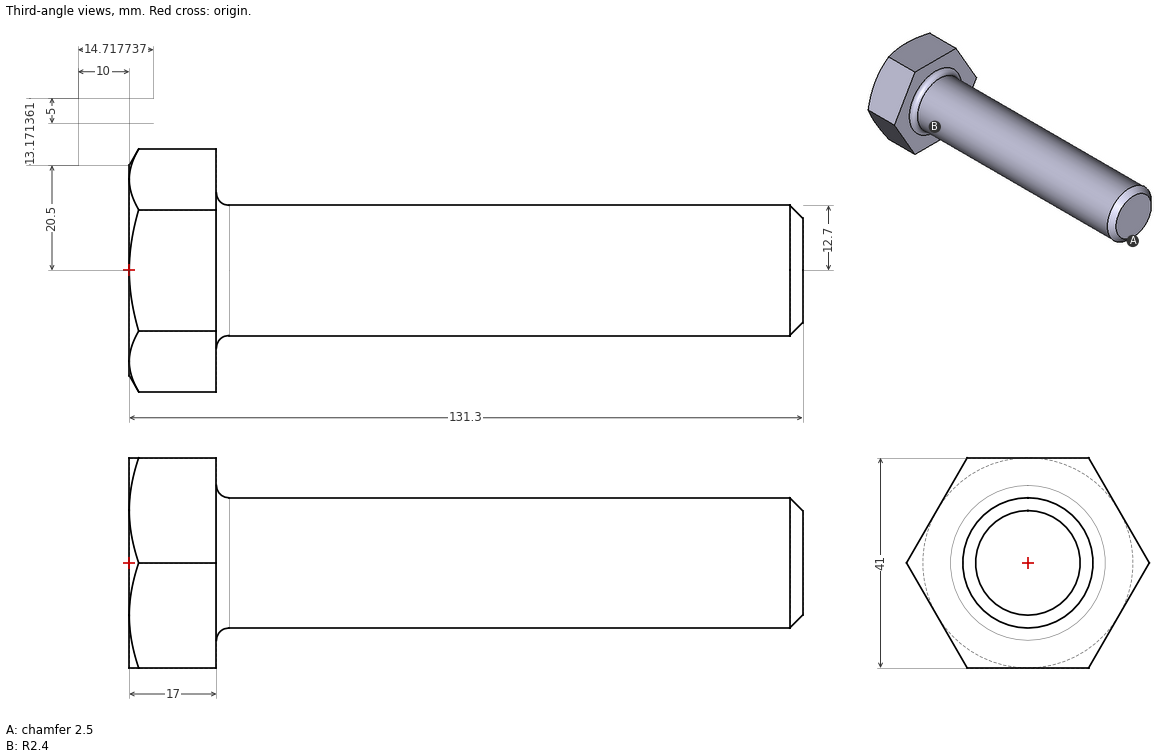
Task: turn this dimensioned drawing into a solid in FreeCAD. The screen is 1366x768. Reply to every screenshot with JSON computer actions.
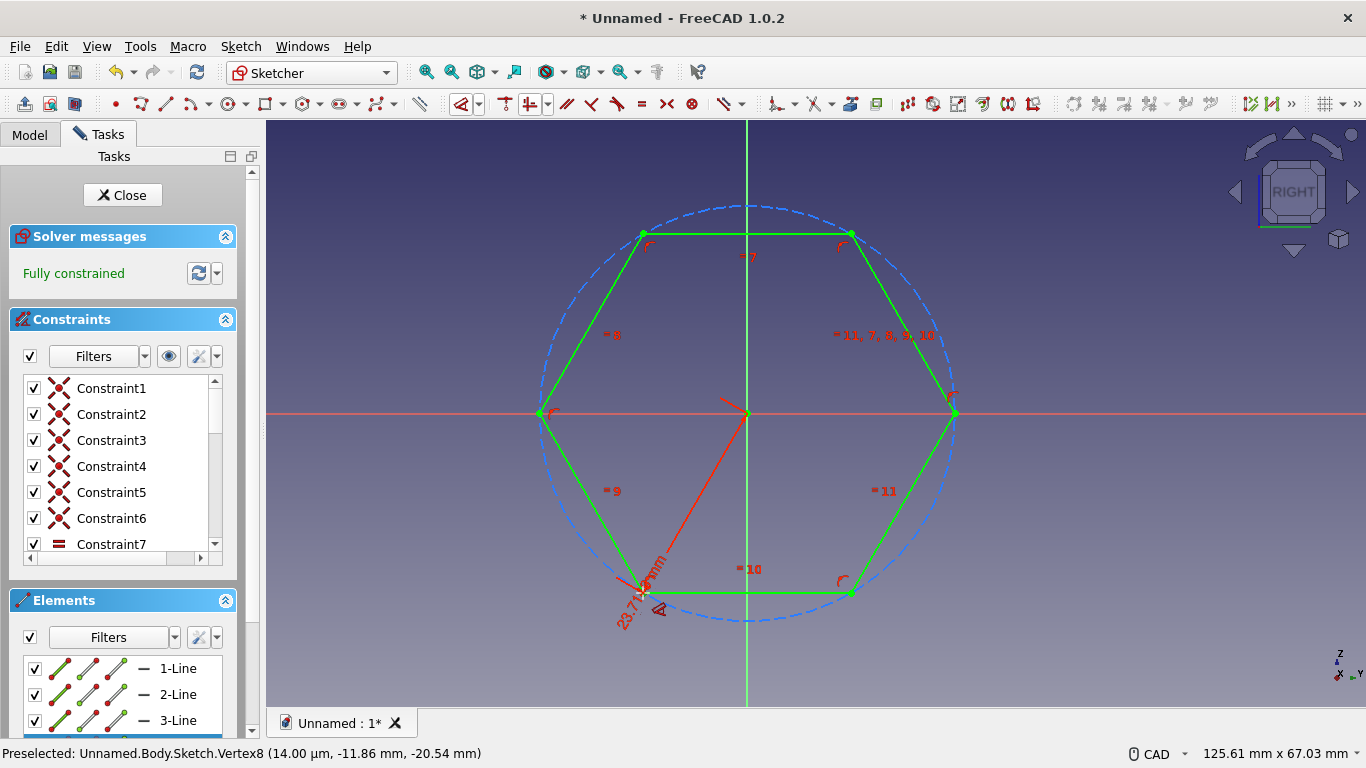
{"action": "left_click", "coordinate": [851, 234]}
{"action": "left_click", "coordinate": [885, 331]}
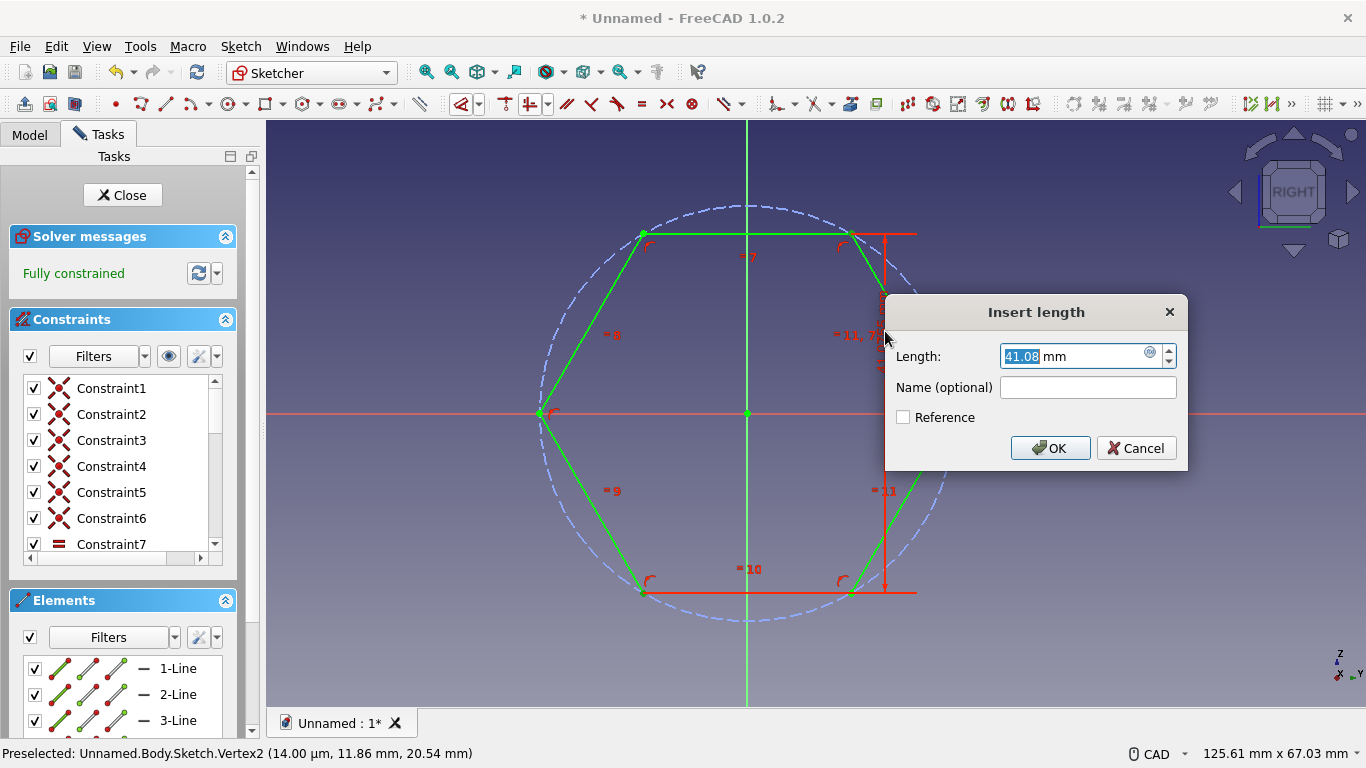
{"action": "type", "text": "41"}
{"action": "key", "text": "Return"}
{"action": "key", "text": "Escape"}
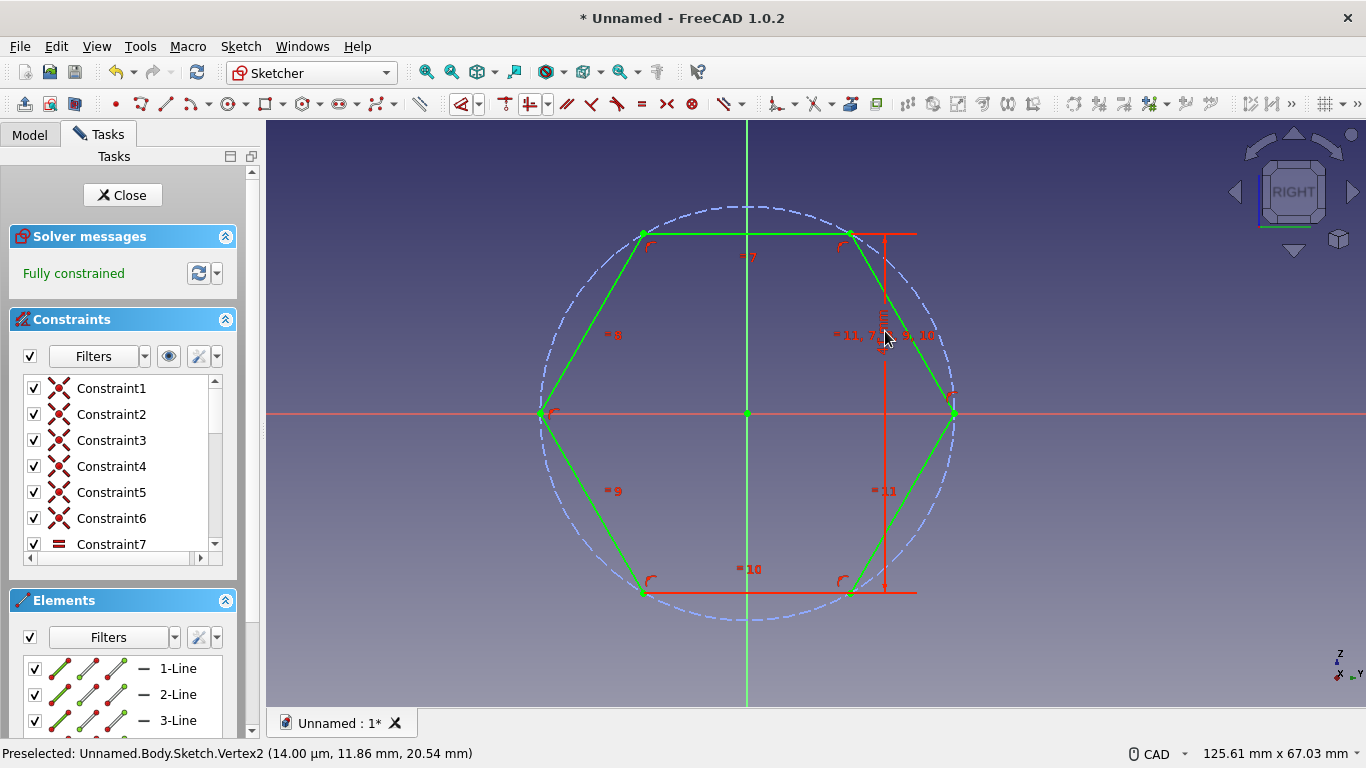
{"action": "left_click", "coordinate": [123, 195]}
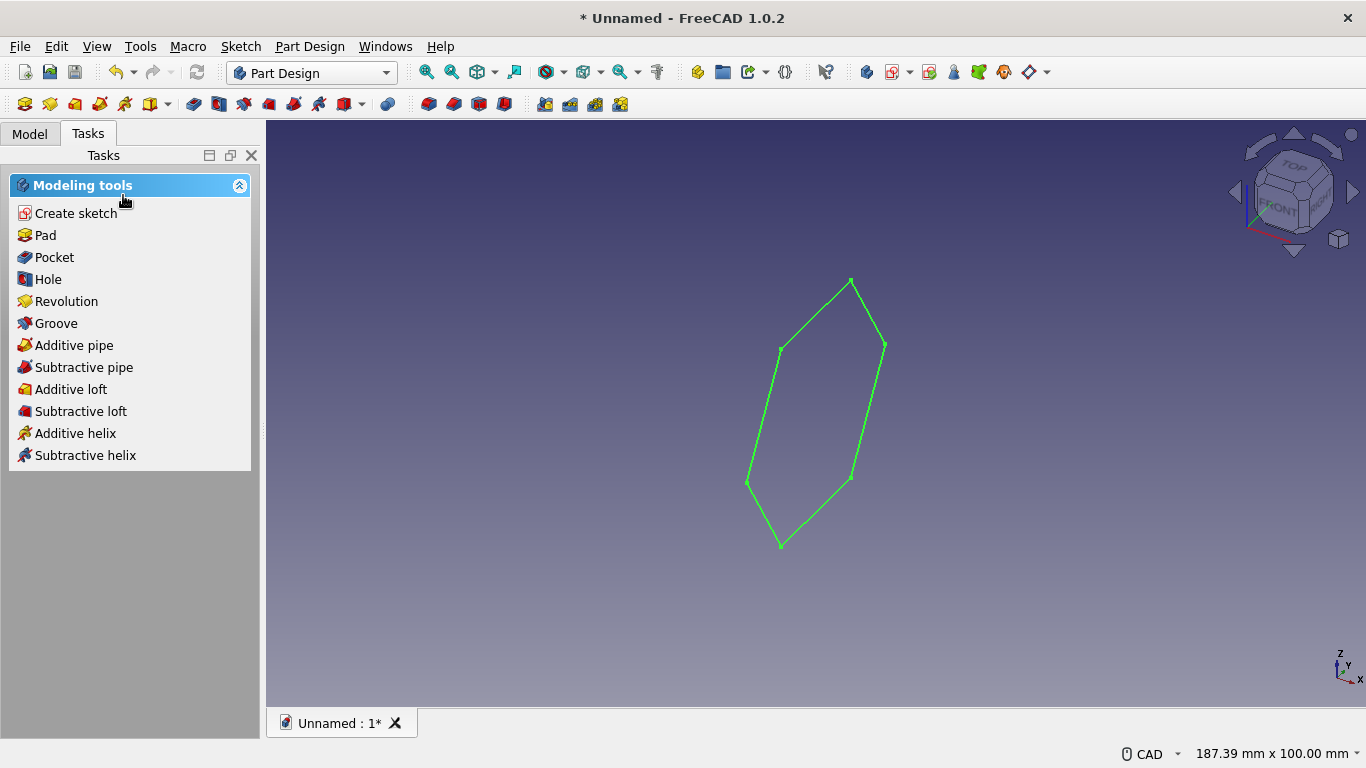
{"action": "left_click", "coordinate": [25, 104]}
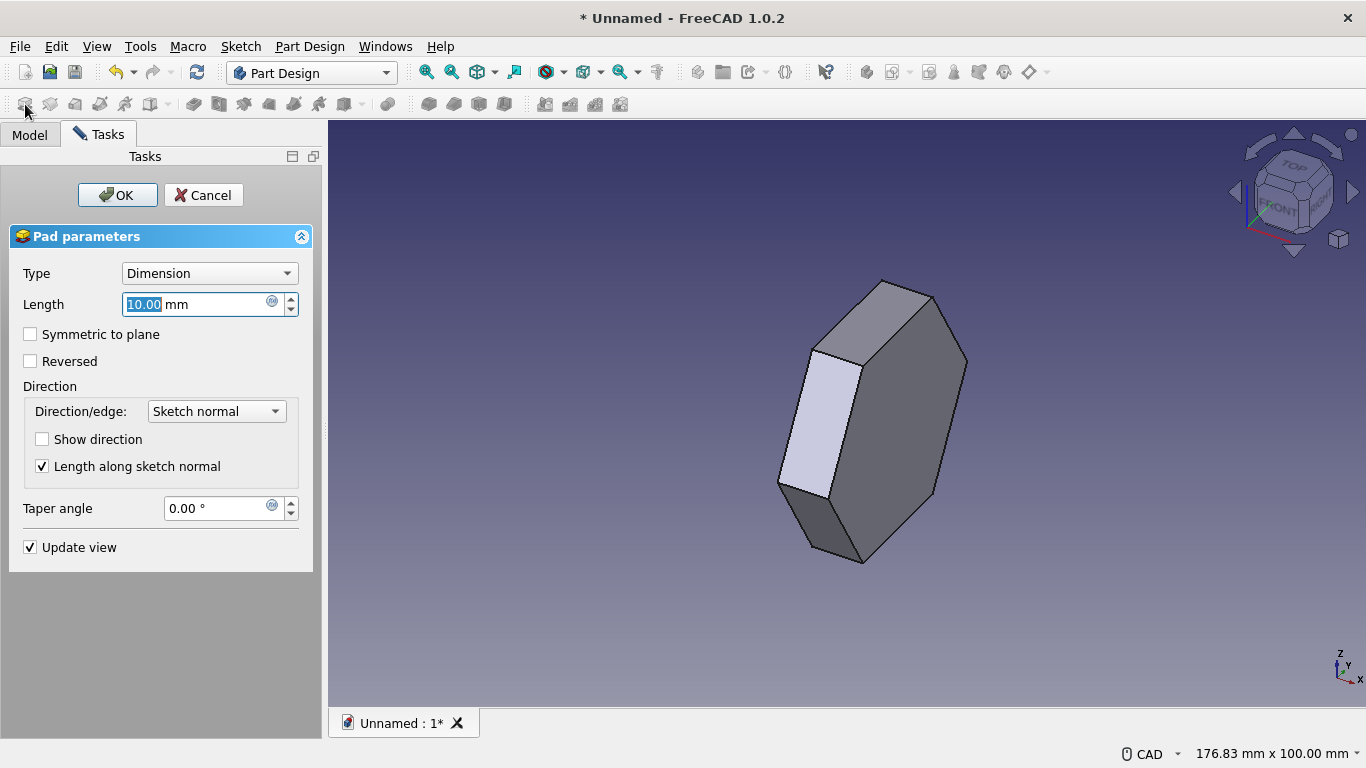
{"action": "type", "text": "17"}
{"action": "key", "text": "Tab"}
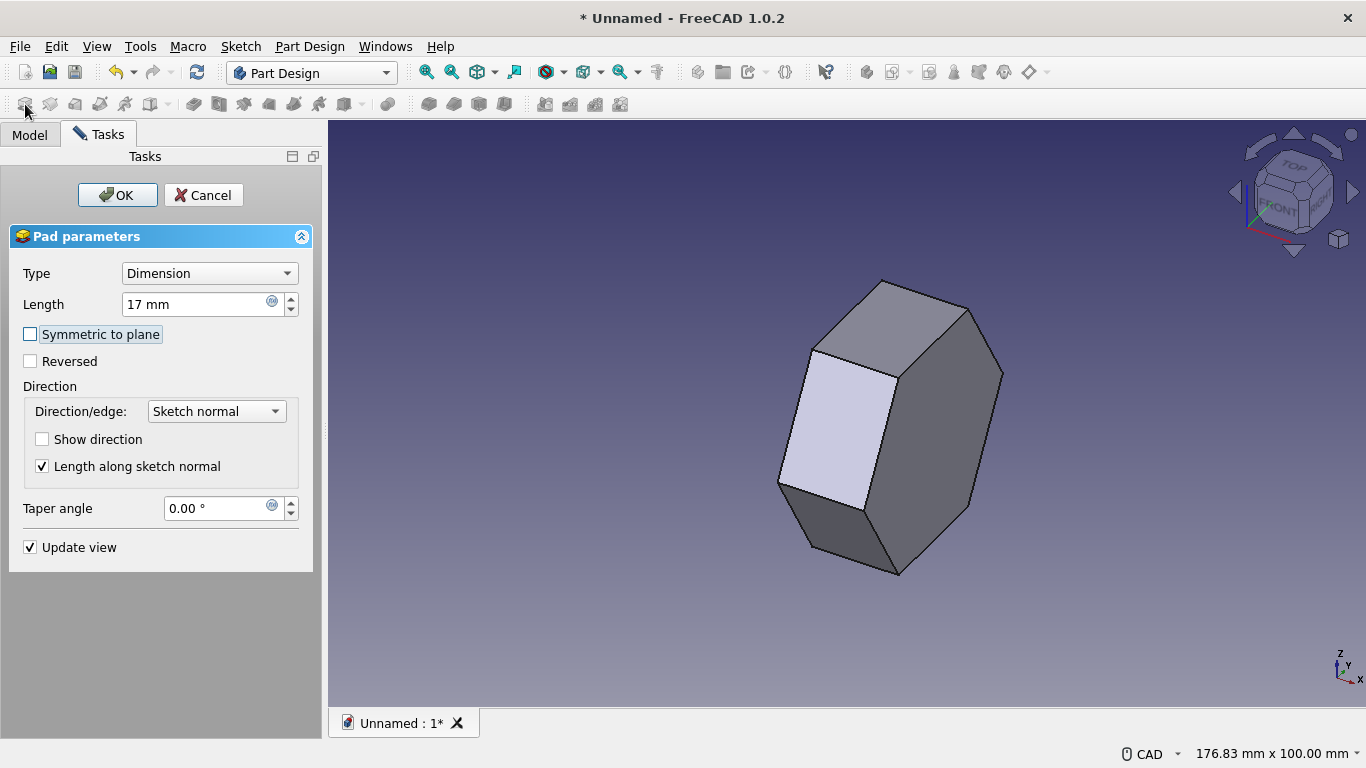
{"action": "left_click", "coordinate": [118, 195]}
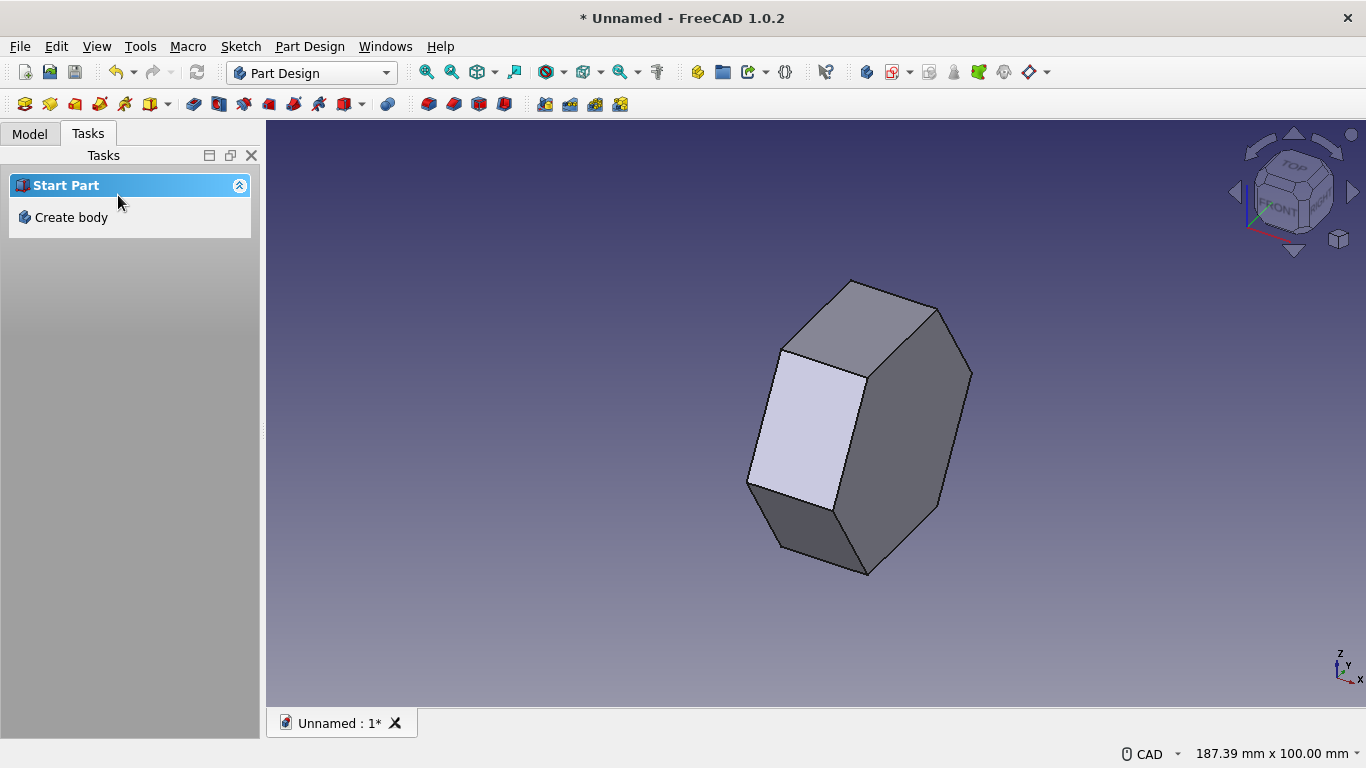
{"action": "left_click", "coordinate": [892, 72]}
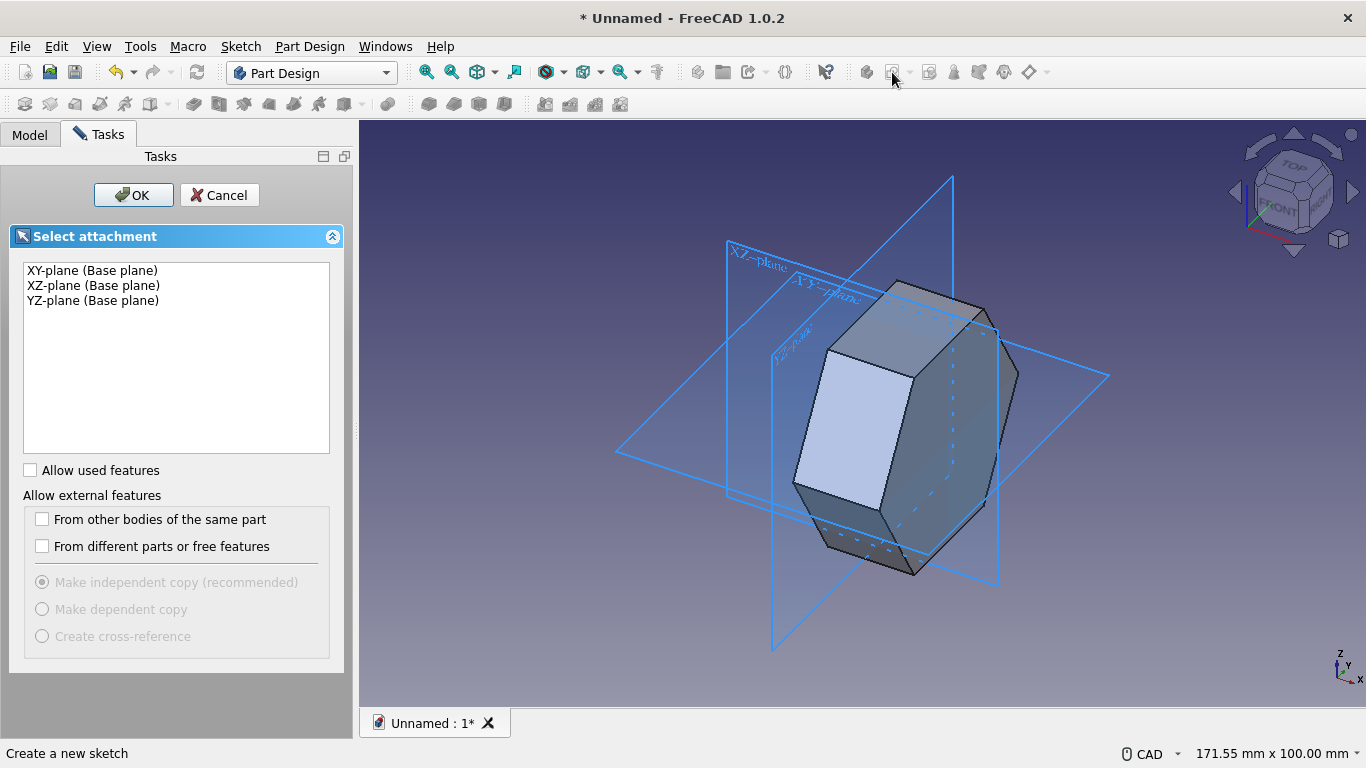
{"action": "left_click", "coordinate": [84, 270]}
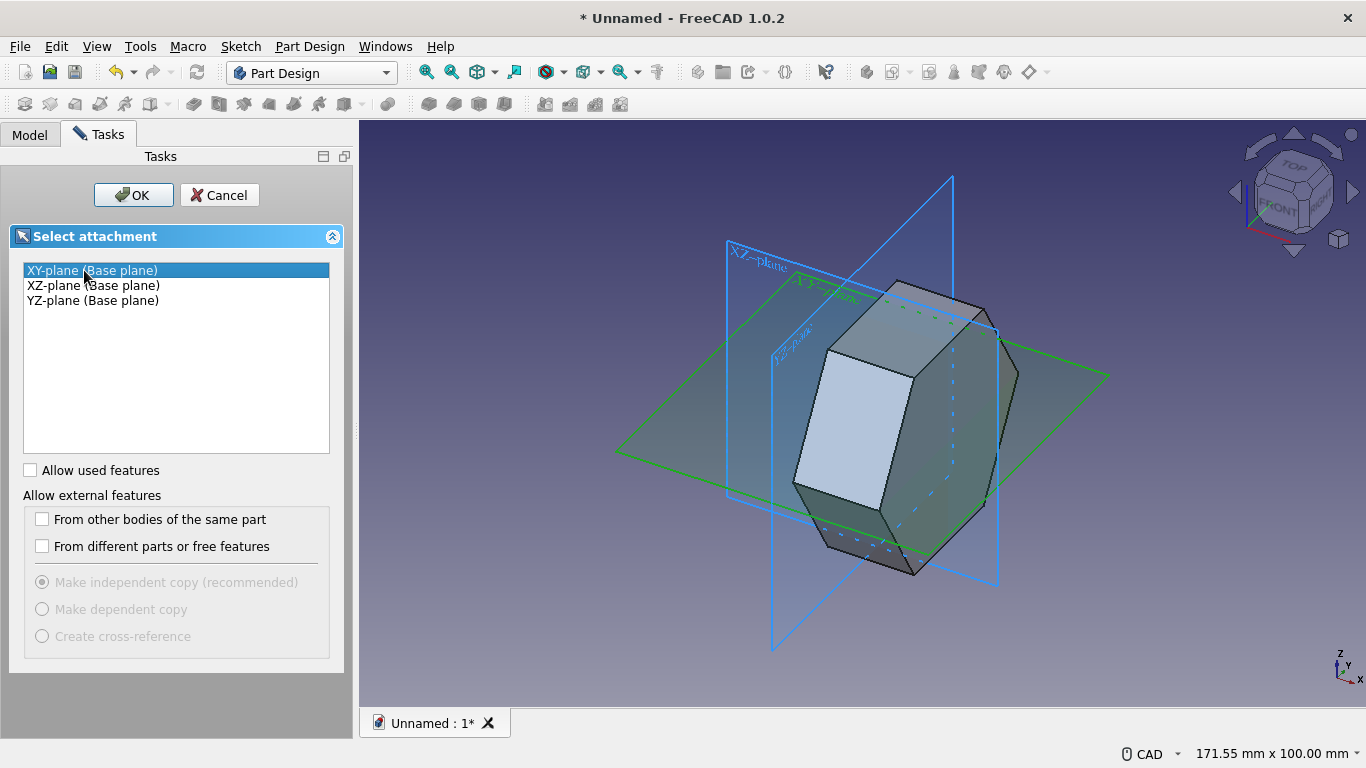
{"action": "left_click", "coordinate": [134, 195]}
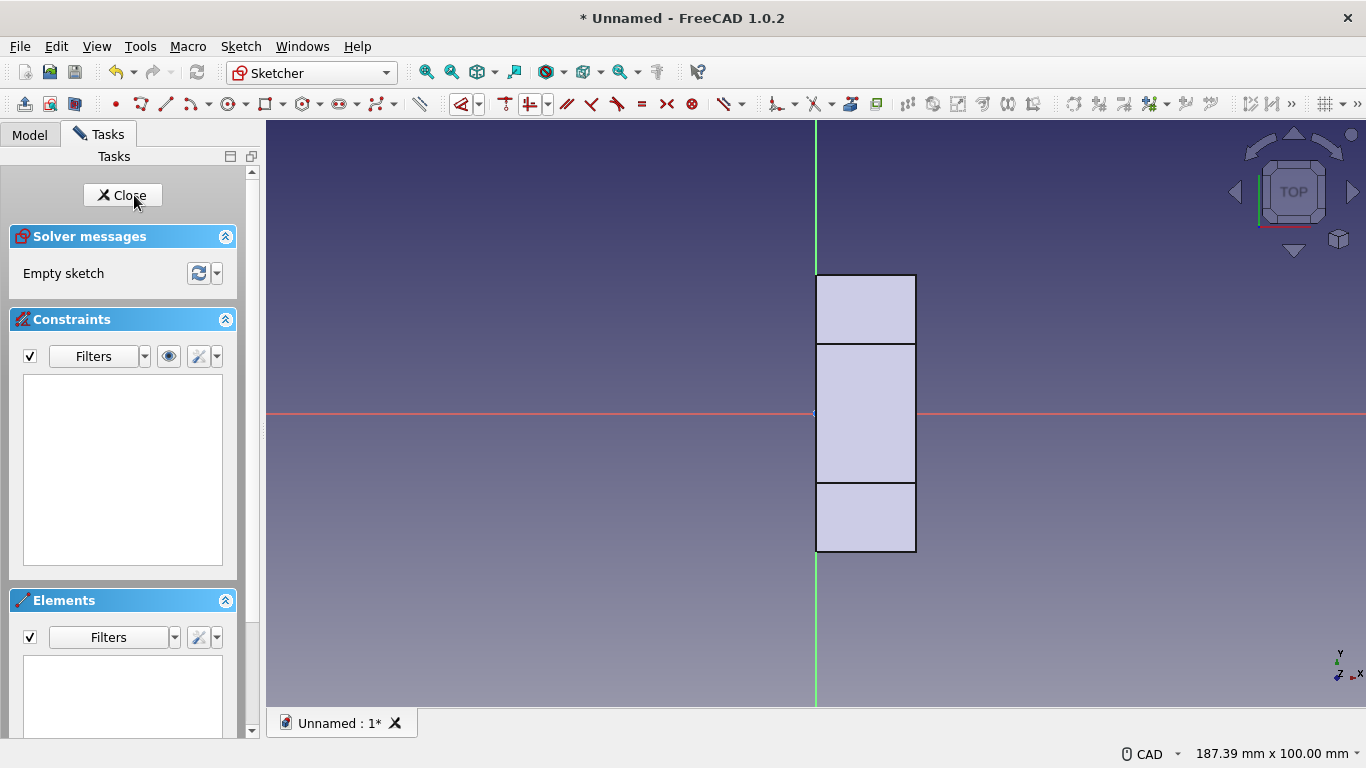
{"action": "key", "text": "q s"}